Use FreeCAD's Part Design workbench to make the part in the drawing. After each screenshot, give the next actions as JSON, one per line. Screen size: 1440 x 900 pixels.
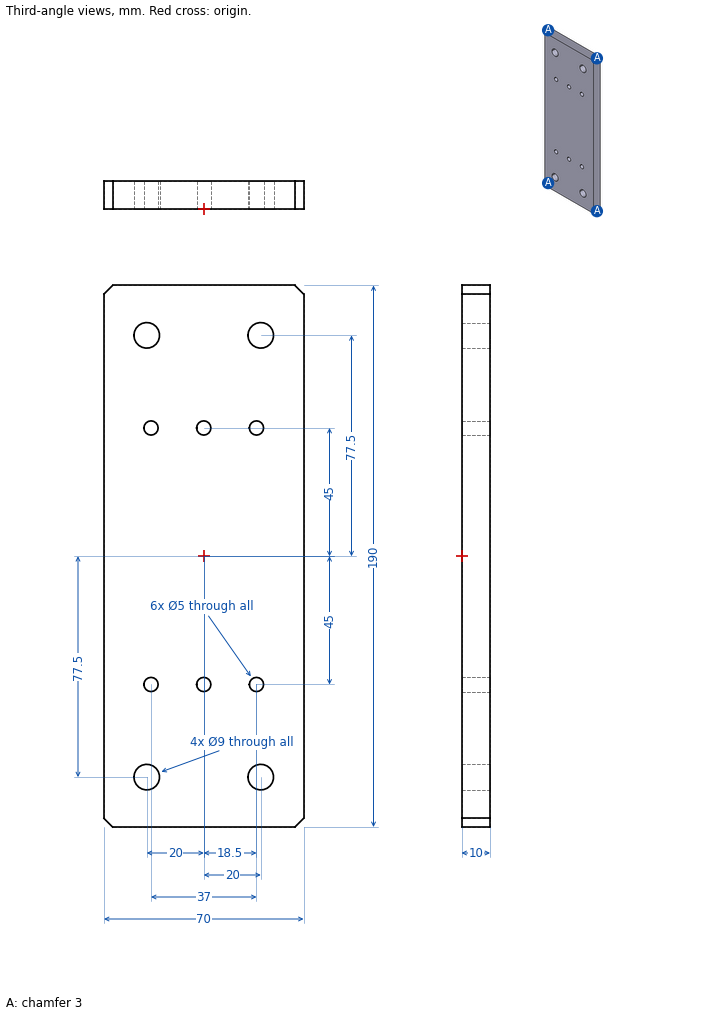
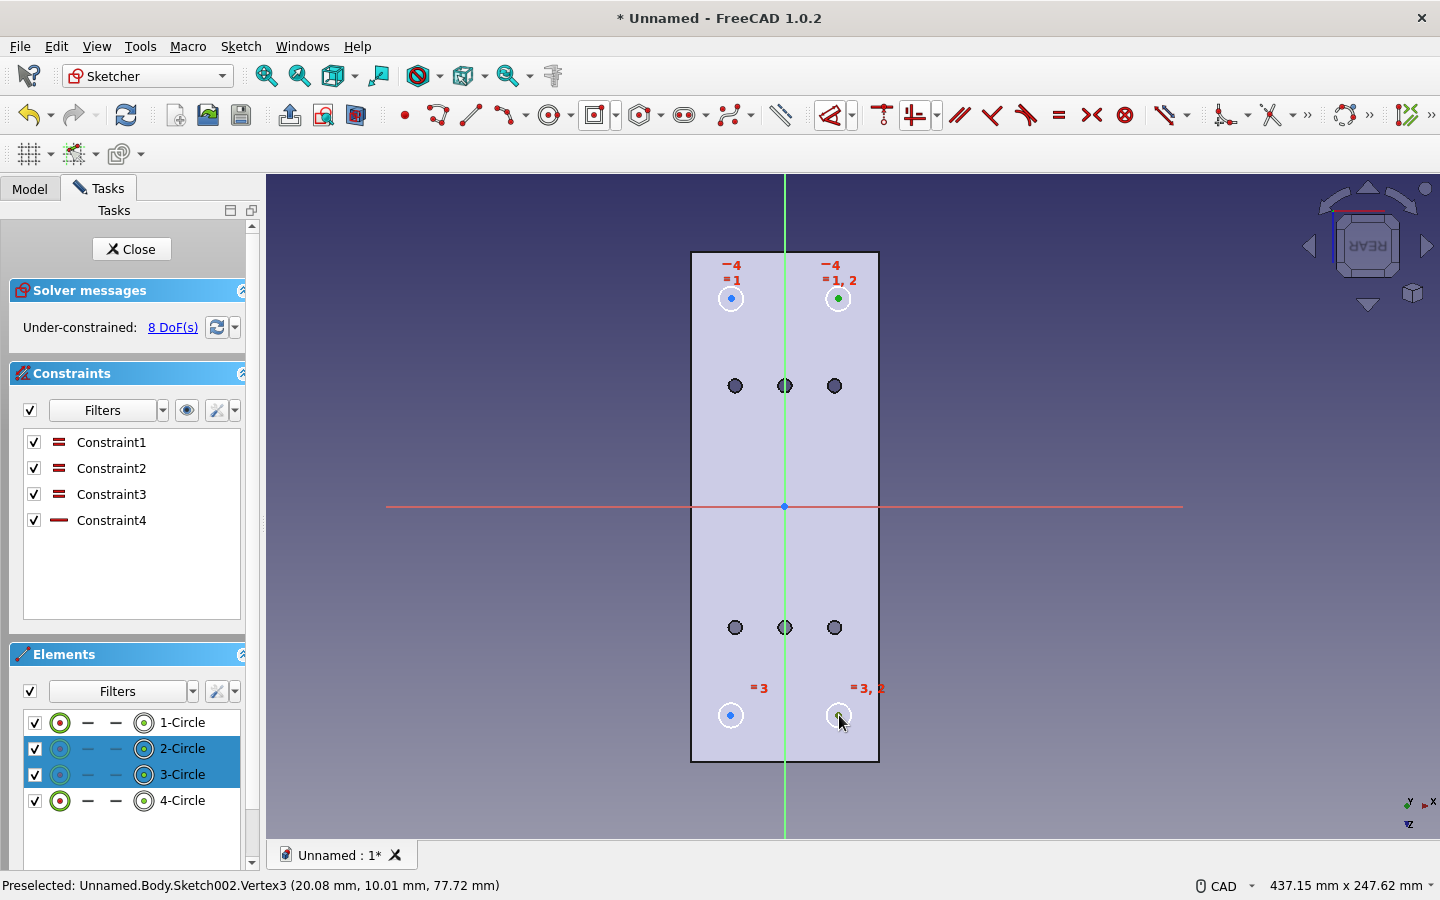
{"action": "key", "text": "v"}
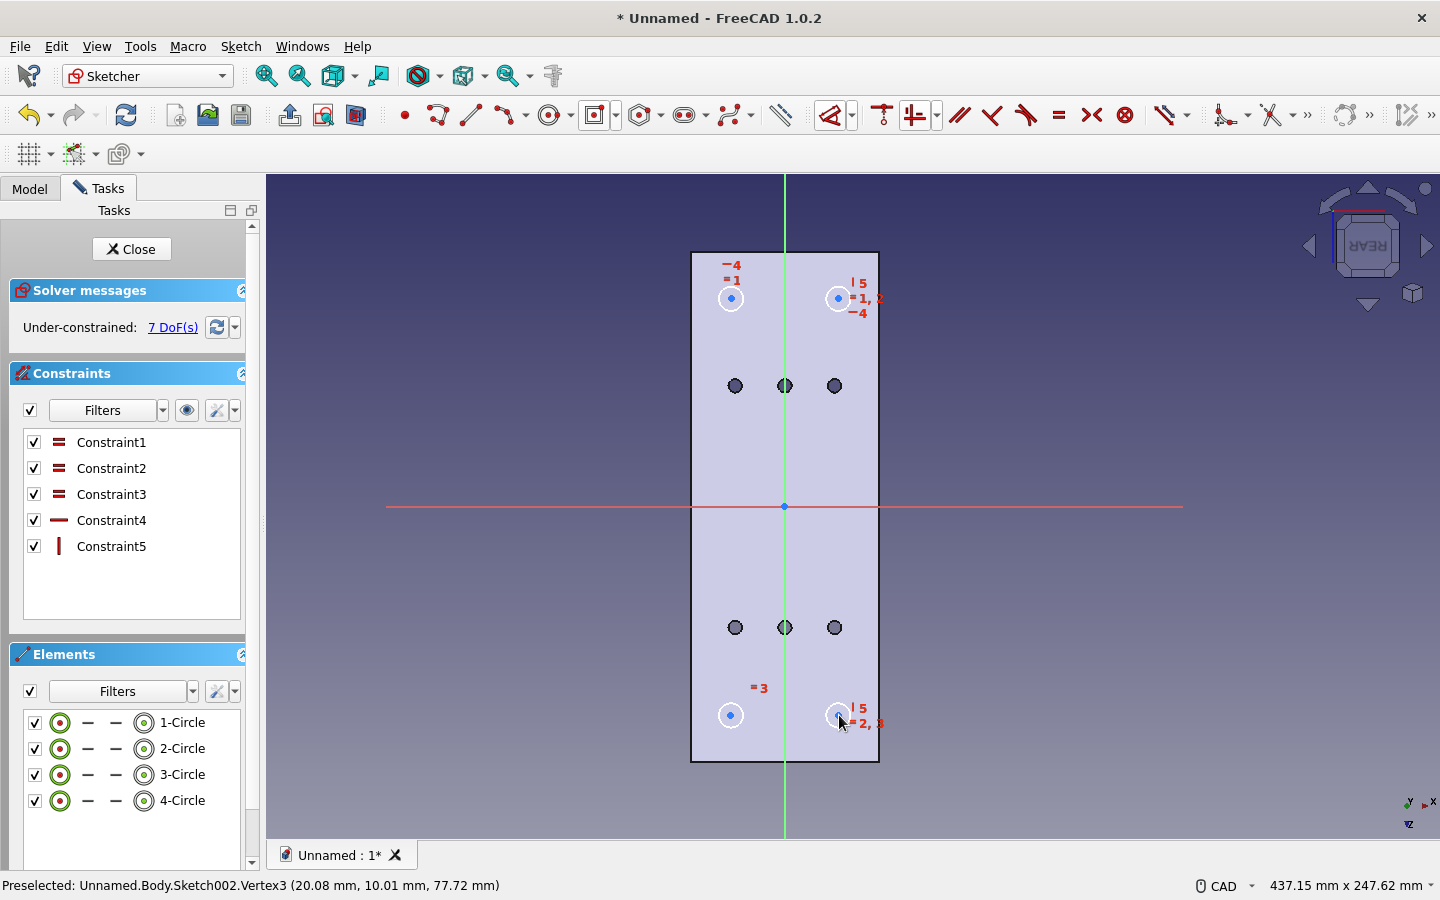
{"action": "left_click", "coordinate": [731, 299]}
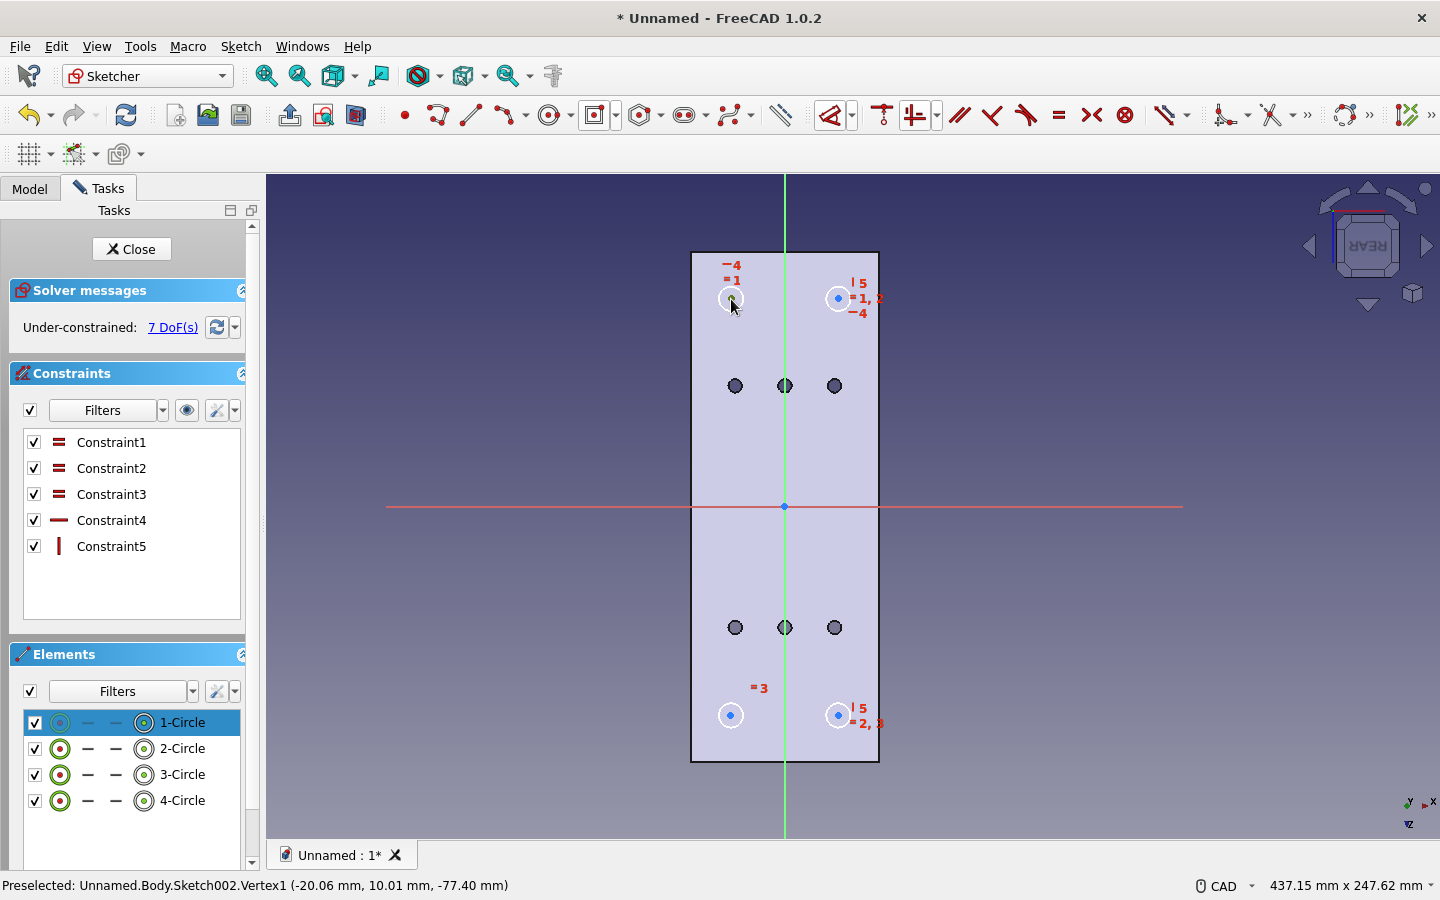
{"action": "left_click", "coordinate": [731, 715]}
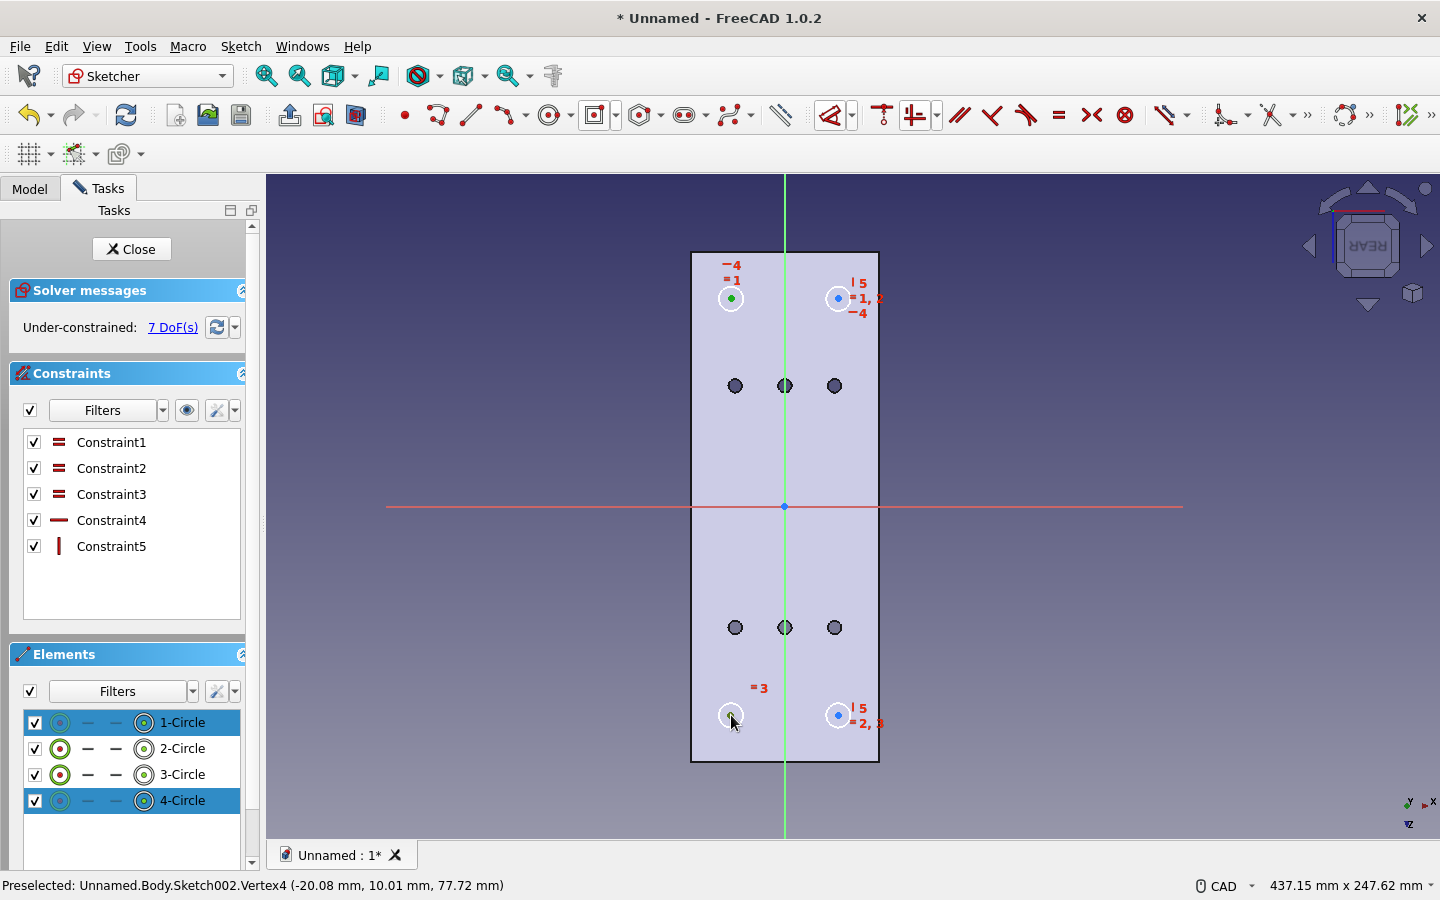
{"action": "key", "text": "v"}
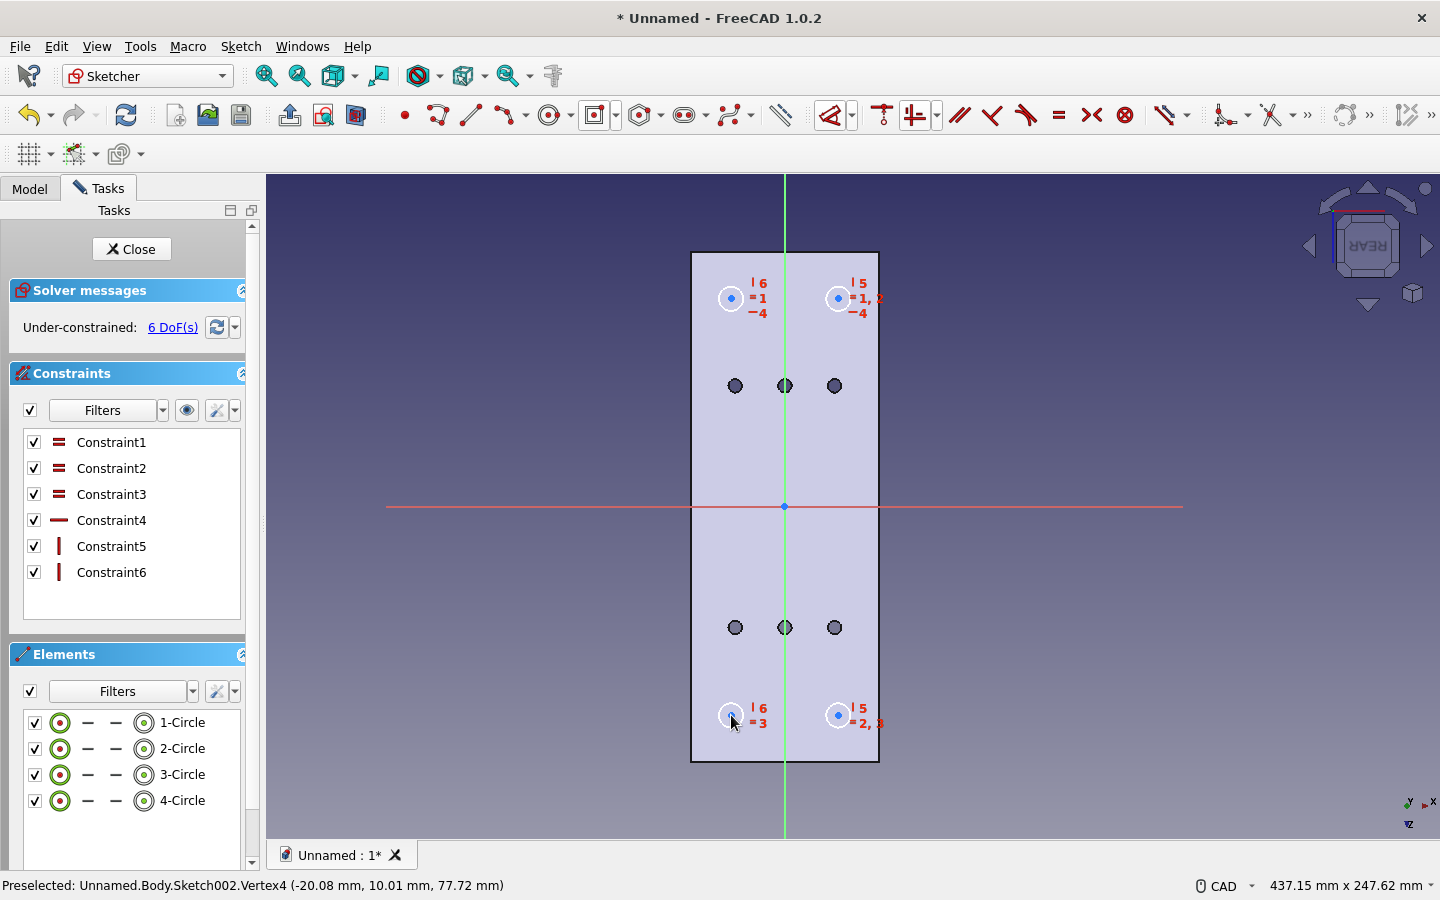
{"action": "left_click", "coordinate": [838, 715]}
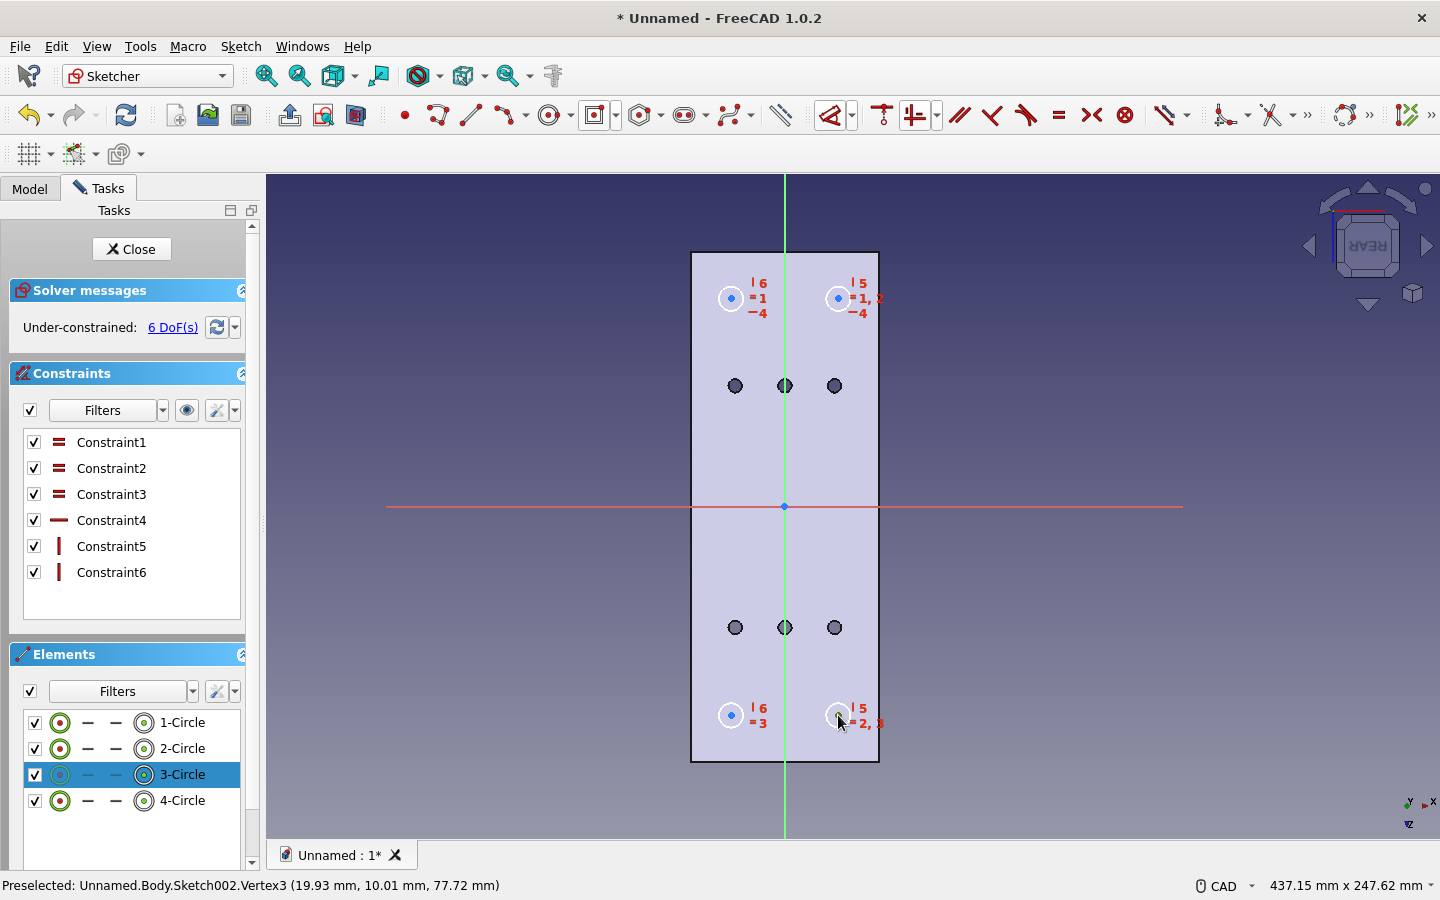
{"action": "left_click", "coordinate": [731, 715]}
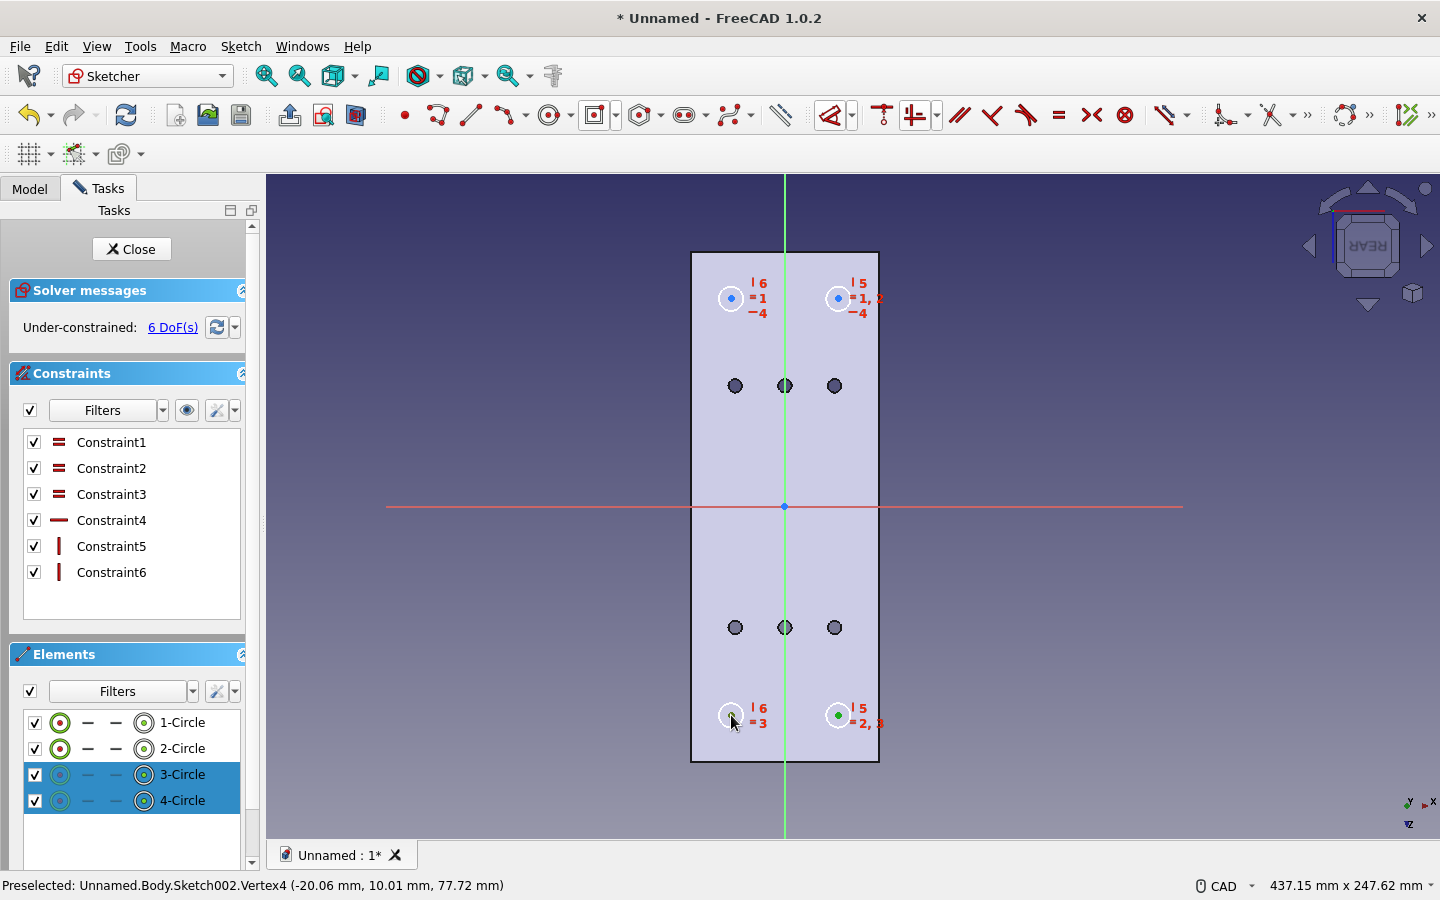
{"action": "key", "text": "h"}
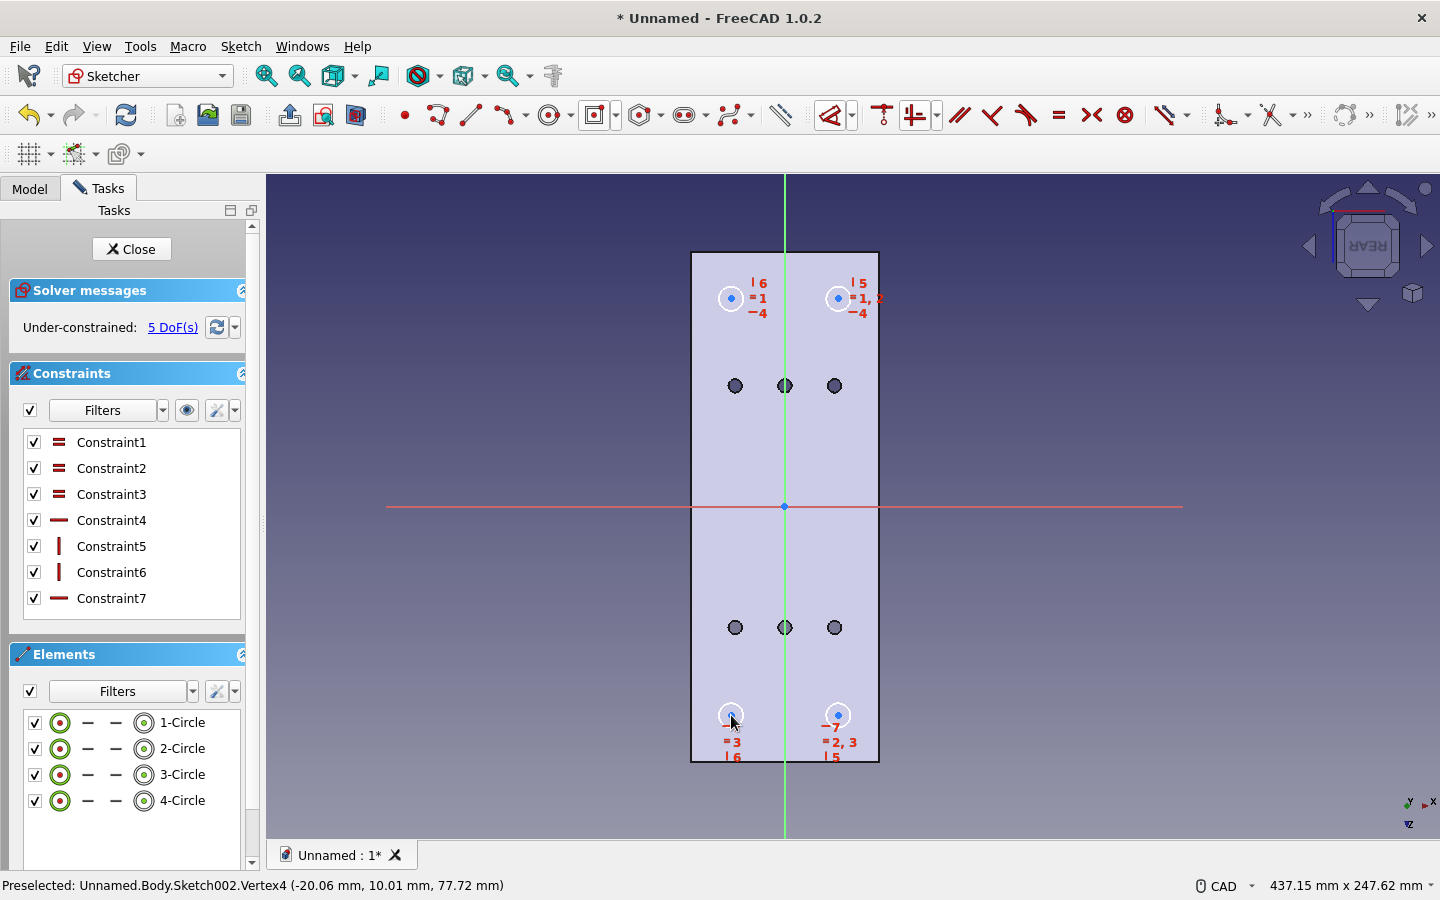
{"action": "scroll", "coordinate": [740, 290], "scroll_direction": "up", "scroll_amount": 3}